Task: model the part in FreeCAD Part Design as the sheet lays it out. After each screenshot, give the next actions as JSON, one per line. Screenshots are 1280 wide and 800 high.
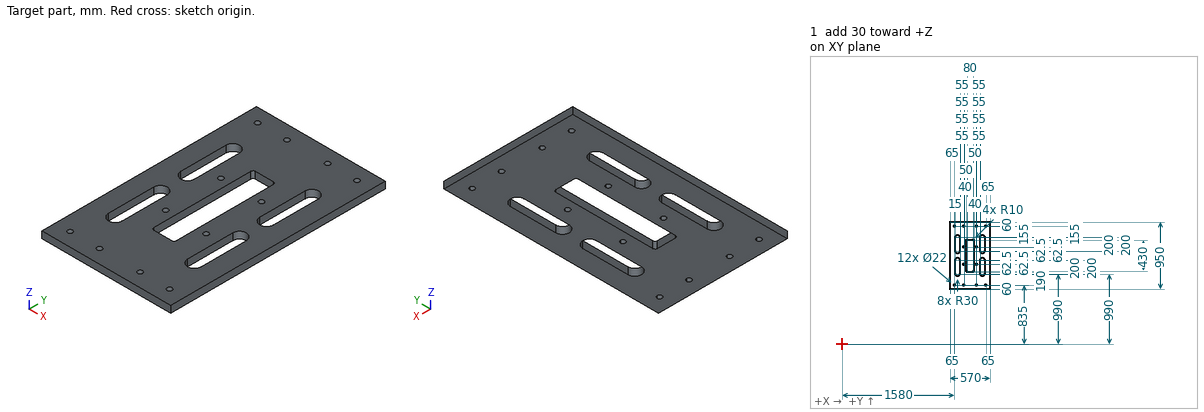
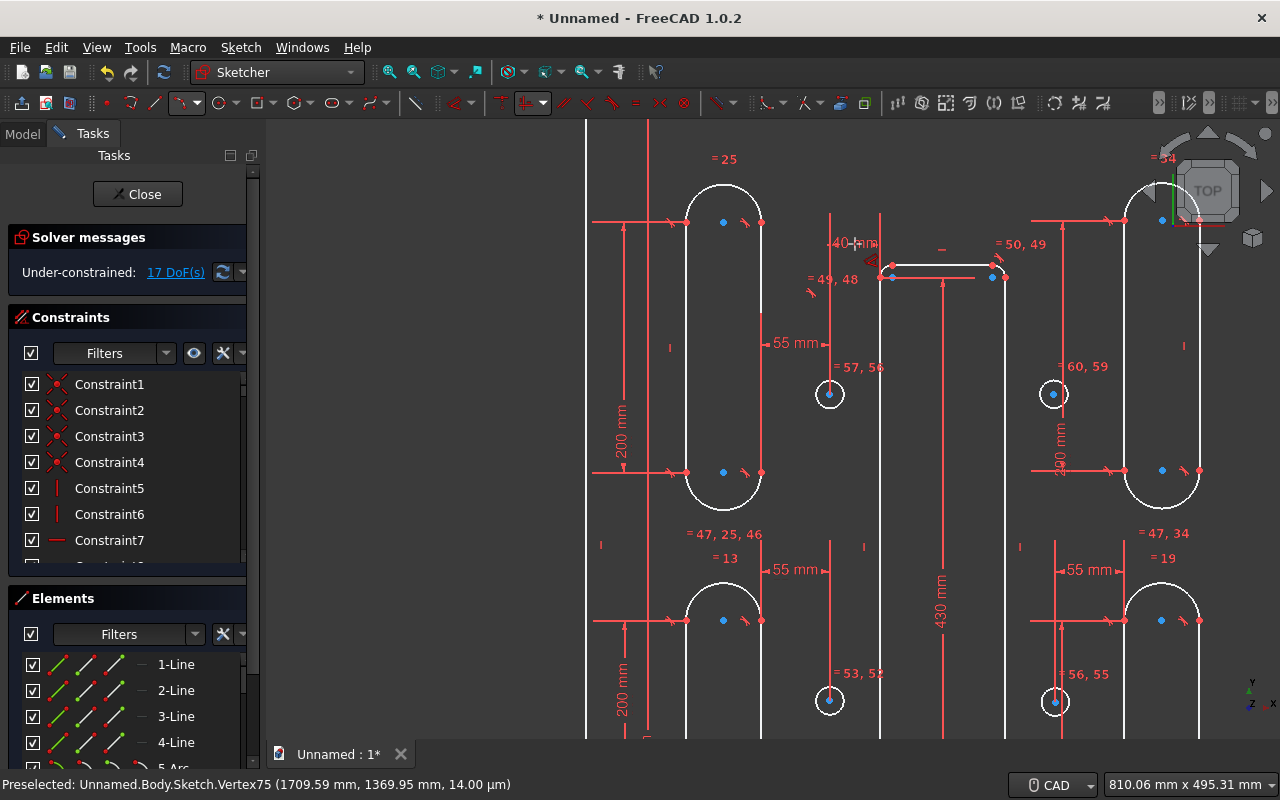
{"action": "scroll", "coordinate": [884, 277], "scroll_direction": "down", "scroll_amount": 8}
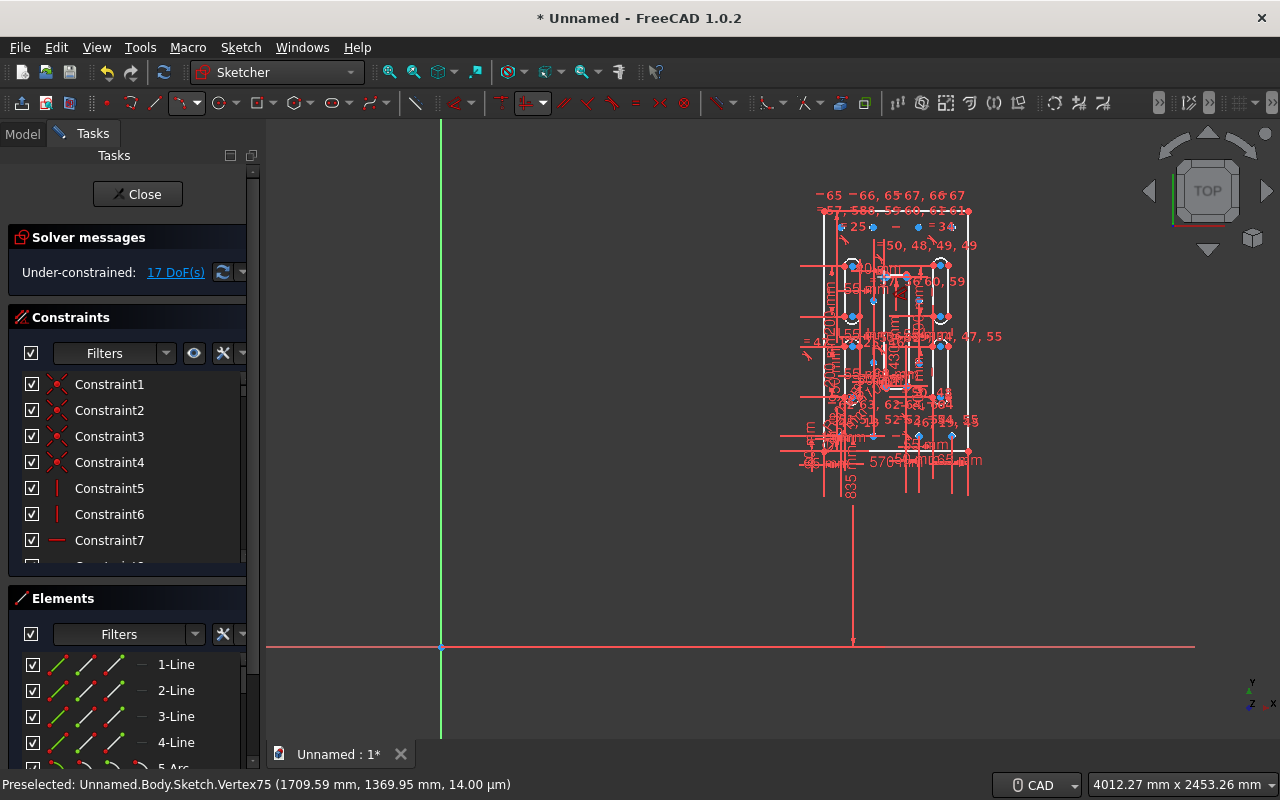
{"action": "scroll", "coordinate": [824, 211], "scroll_direction": "up", "scroll_amount": 5}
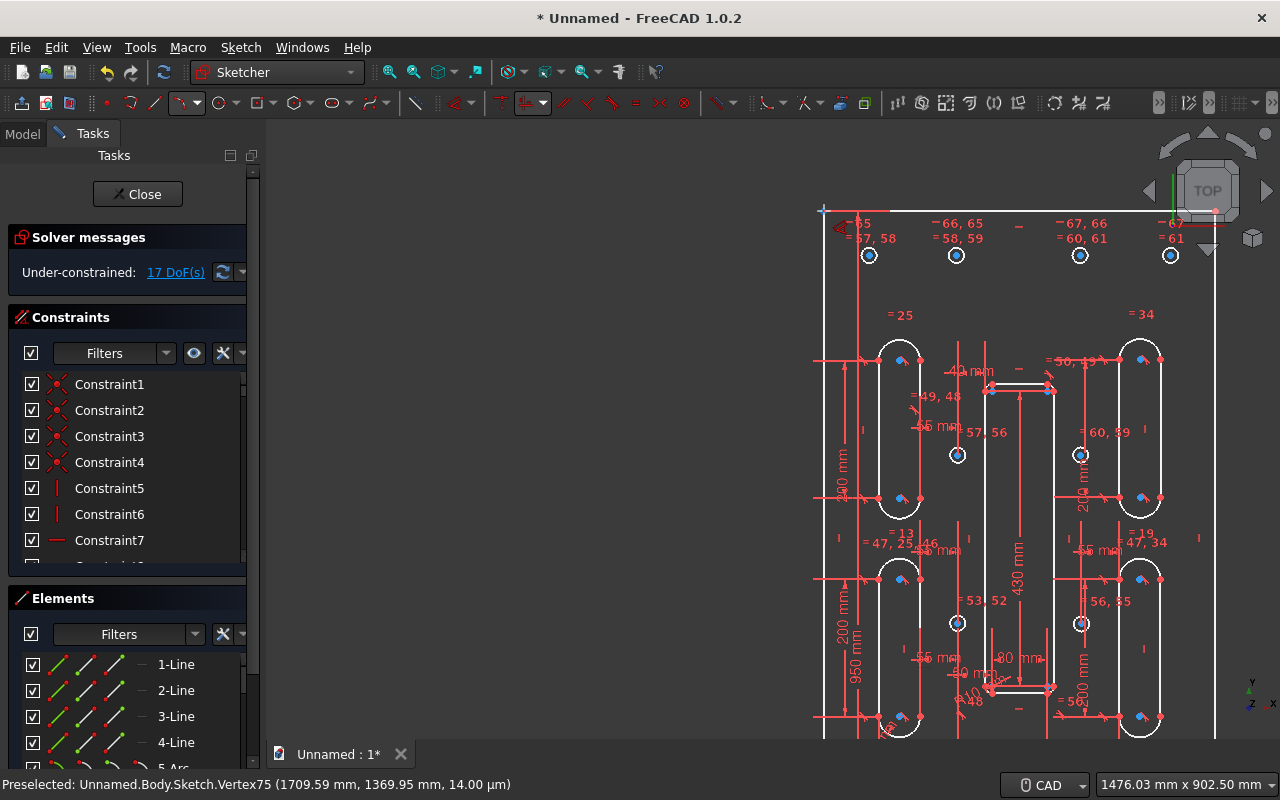
{"action": "left_click", "coordinate": [824, 211]}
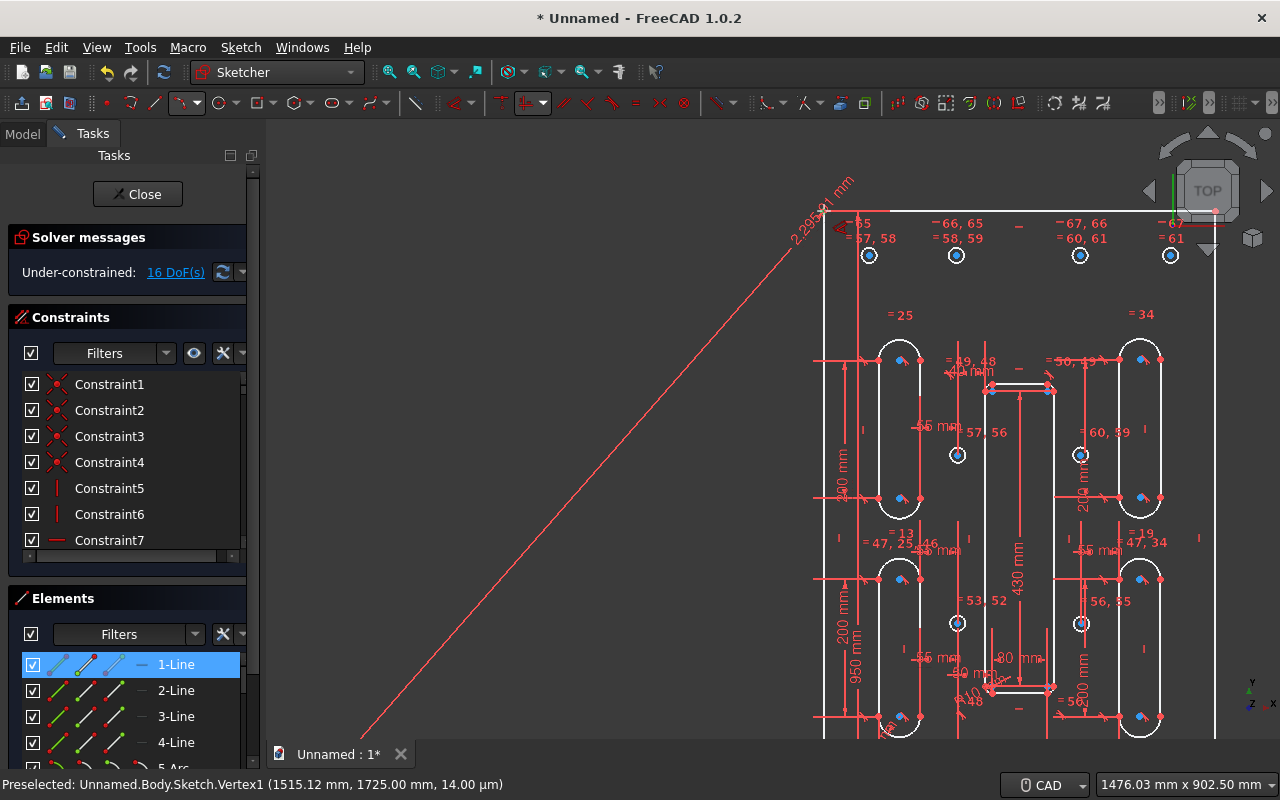
{"action": "left_click", "coordinate": [869, 255]}
{"action": "left_click", "coordinate": [846, 177]}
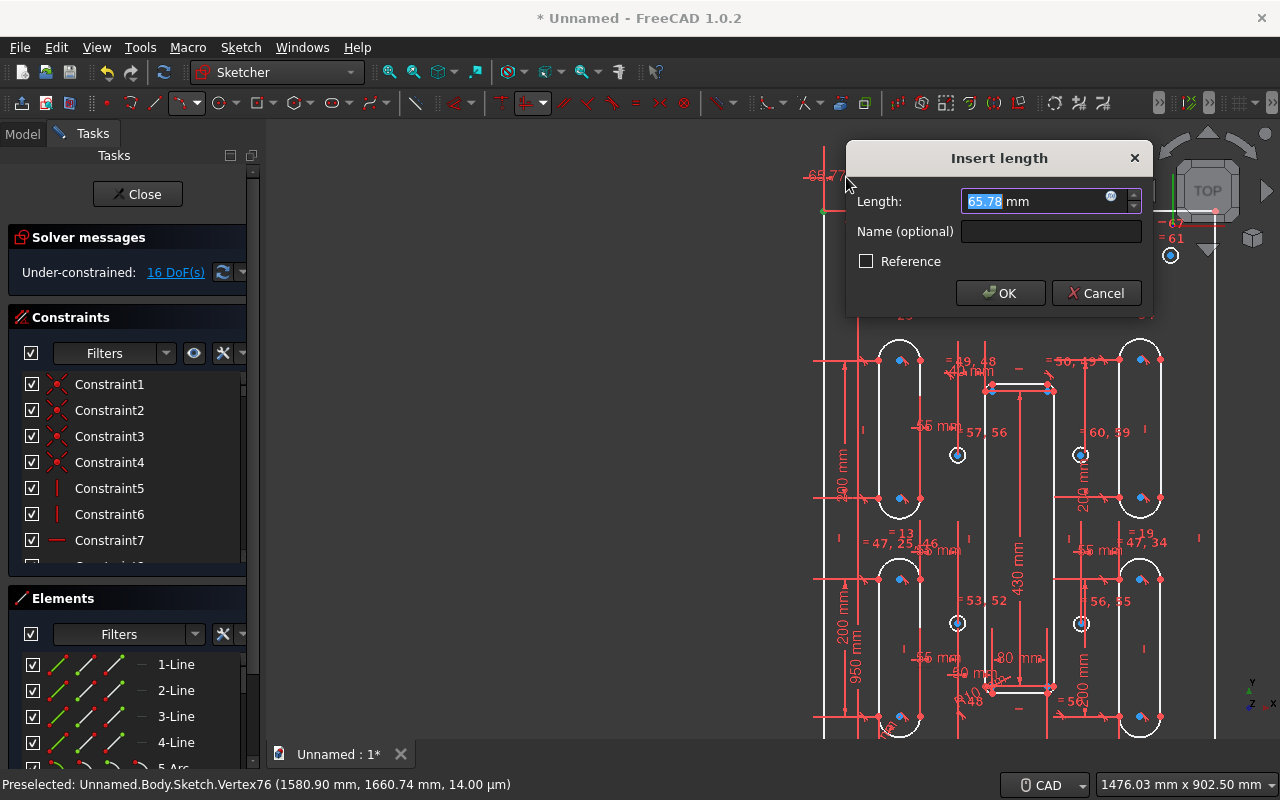
{"action": "type", "text": "65"}
{"action": "key", "text": "Return"}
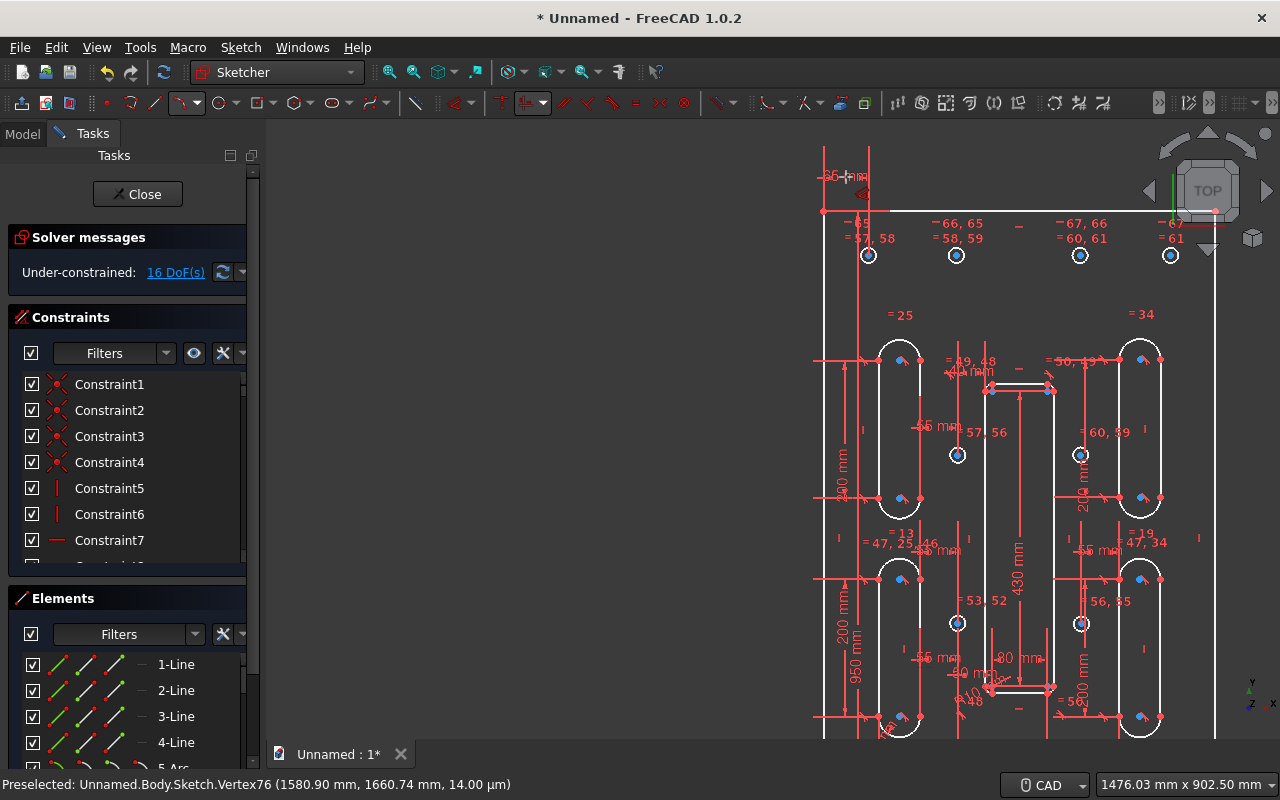
{"action": "left_click", "coordinate": [824, 211]}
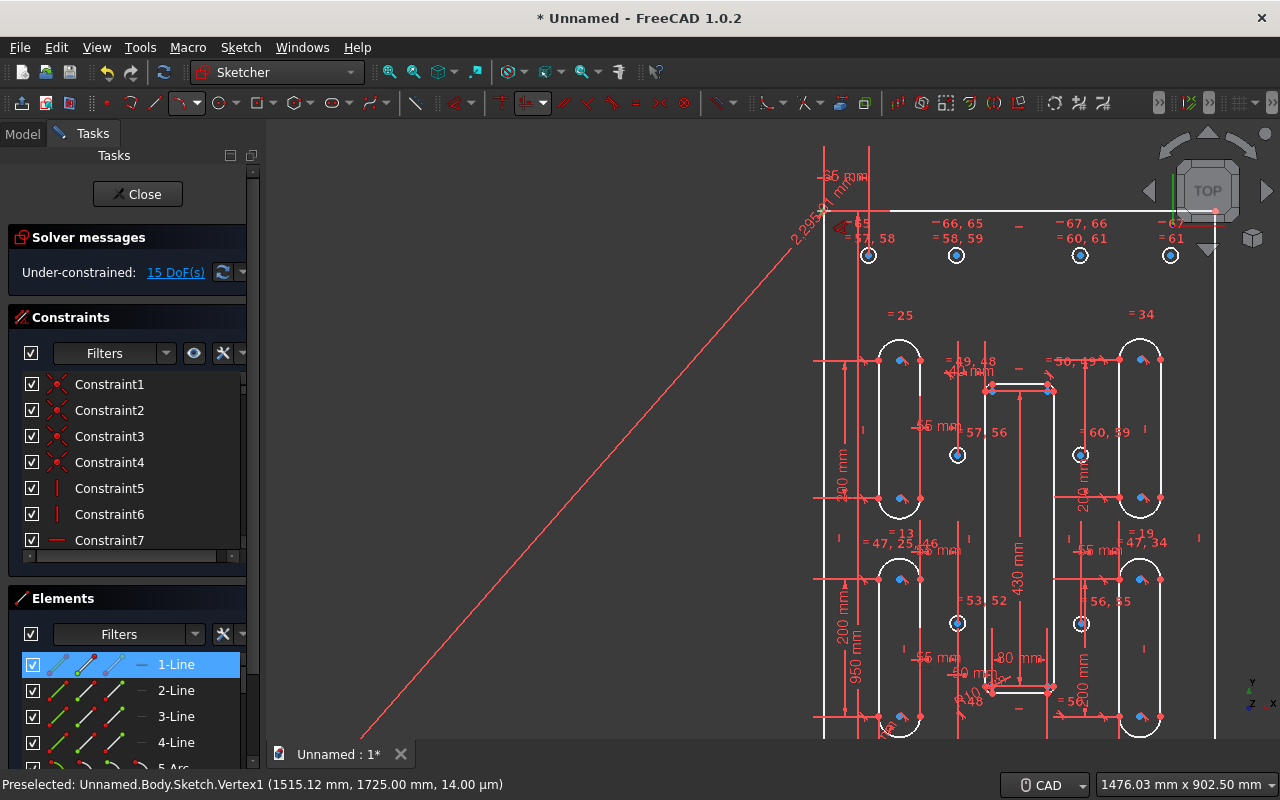
{"action": "left_click", "coordinate": [869, 255]}
{"action": "left_click", "coordinate": [903, 233]}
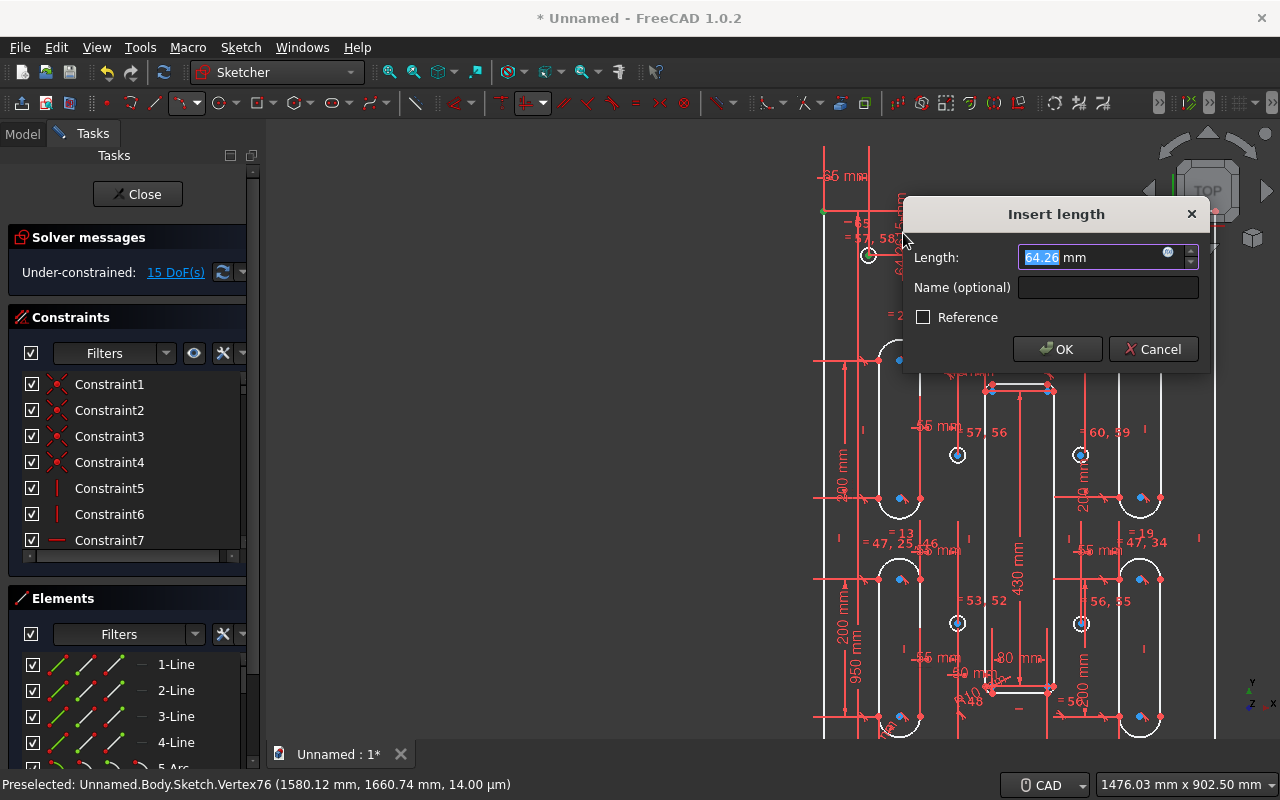
{"action": "type", "text": "60"}
{"action": "key", "text": "Return"}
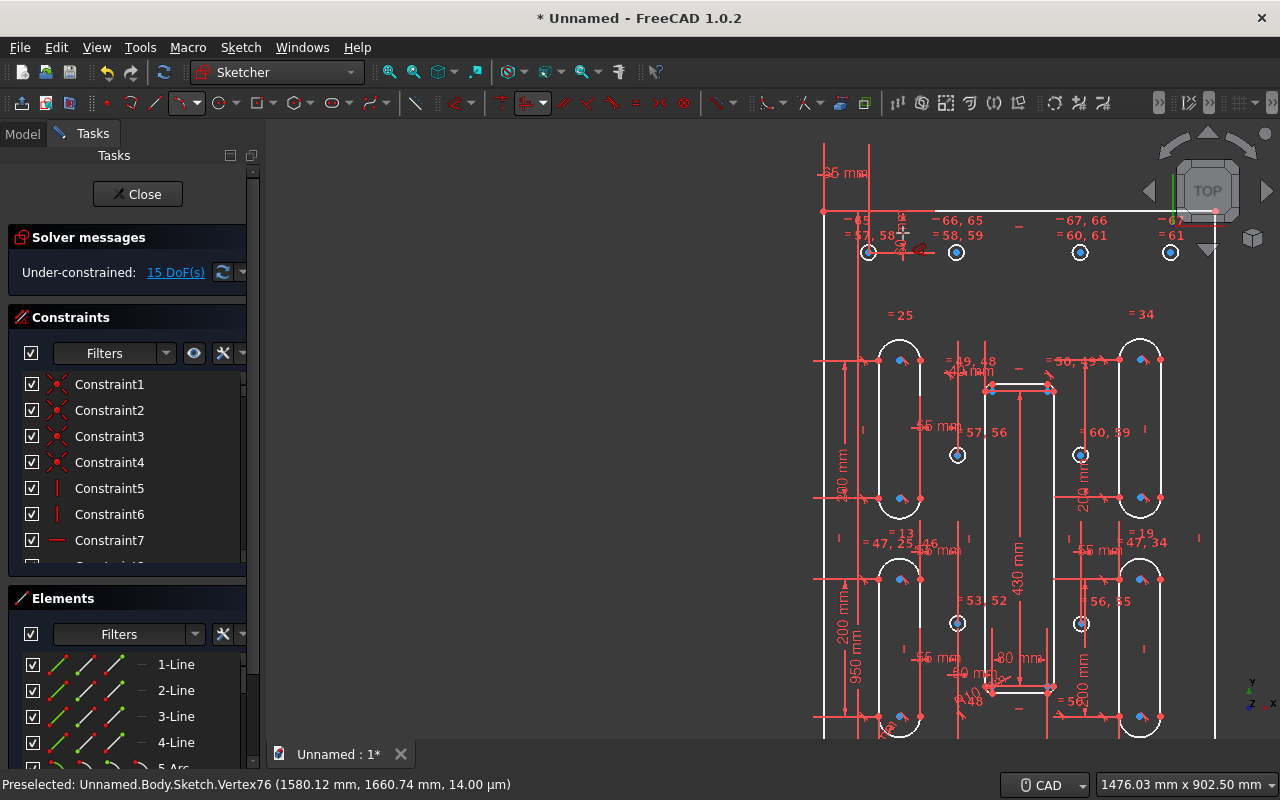
{"action": "left_click", "coordinate": [920, 361]}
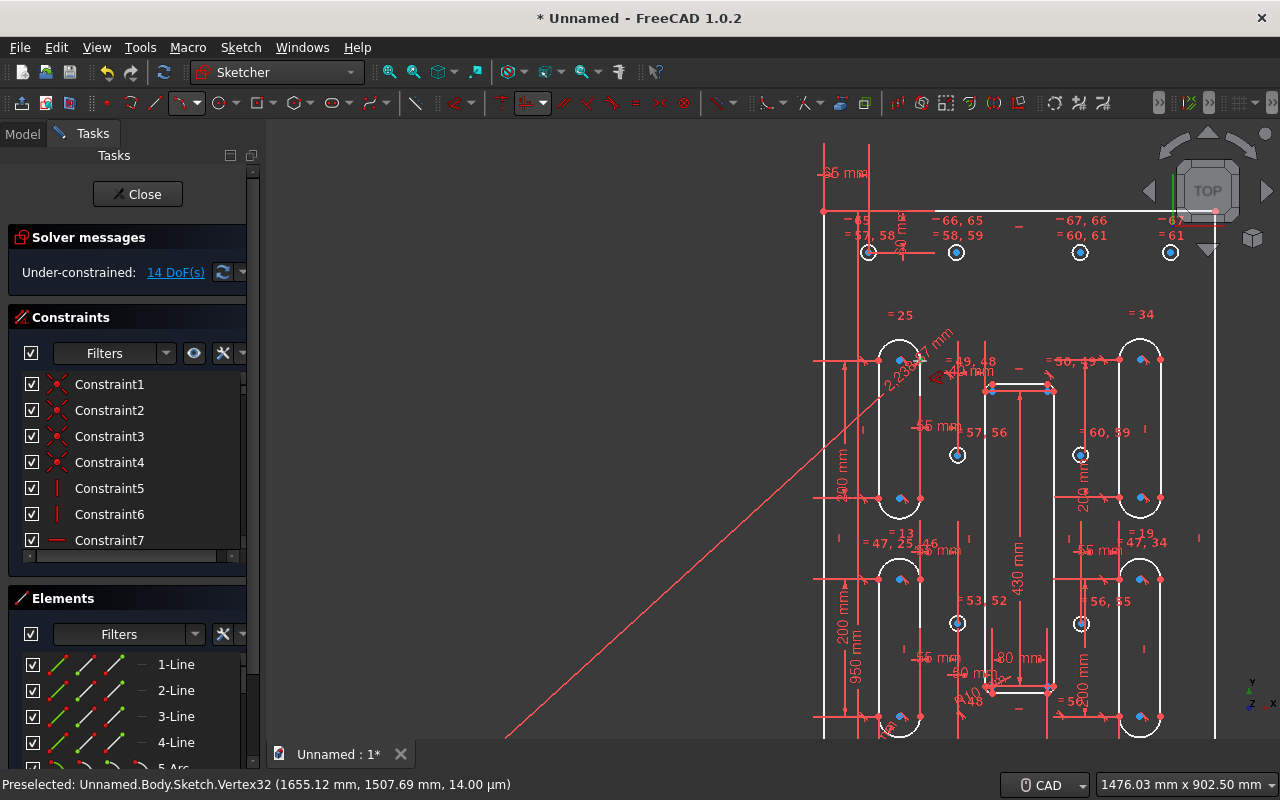
{"action": "left_click", "coordinate": [956, 253]}
{"action": "left_click", "coordinate": [938, 395]}